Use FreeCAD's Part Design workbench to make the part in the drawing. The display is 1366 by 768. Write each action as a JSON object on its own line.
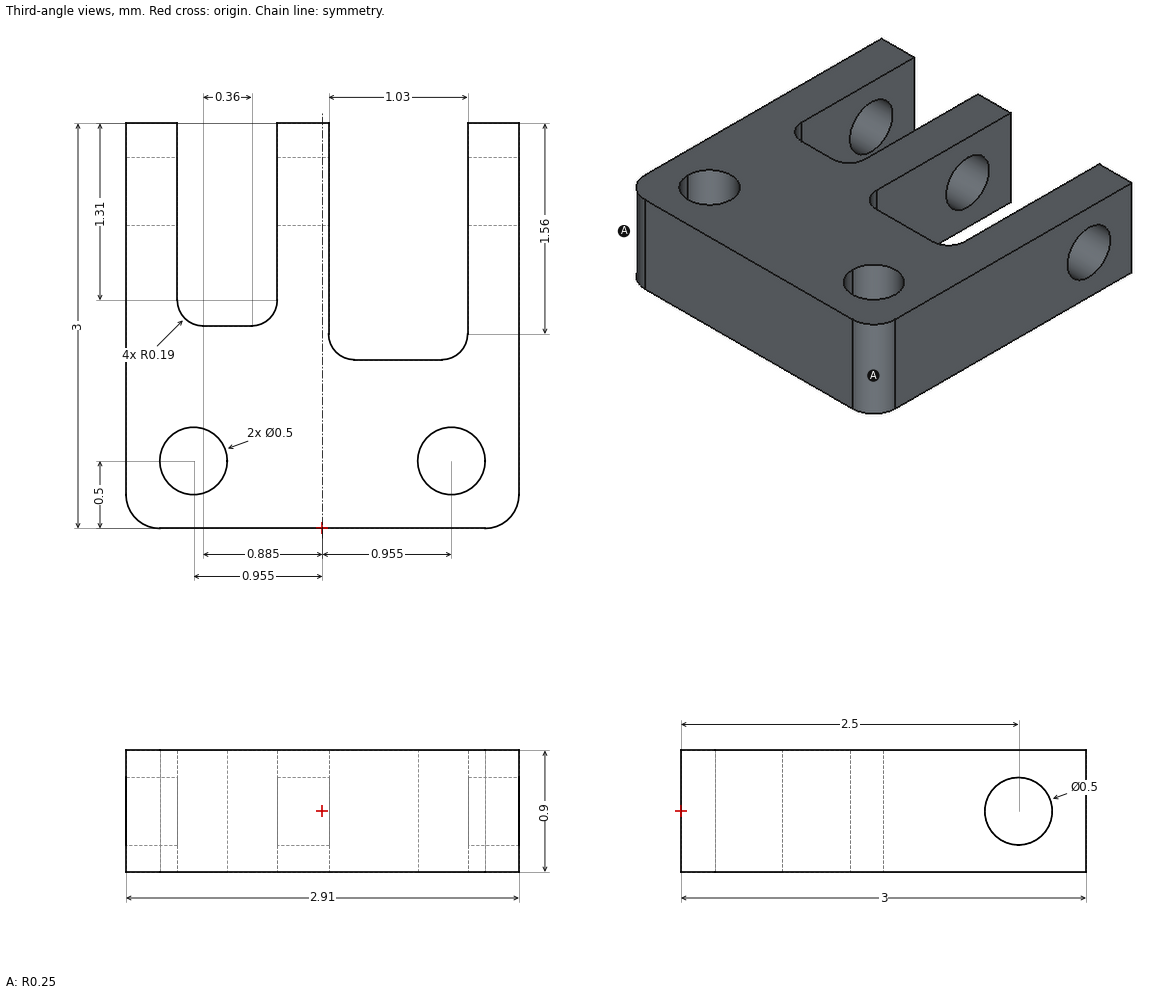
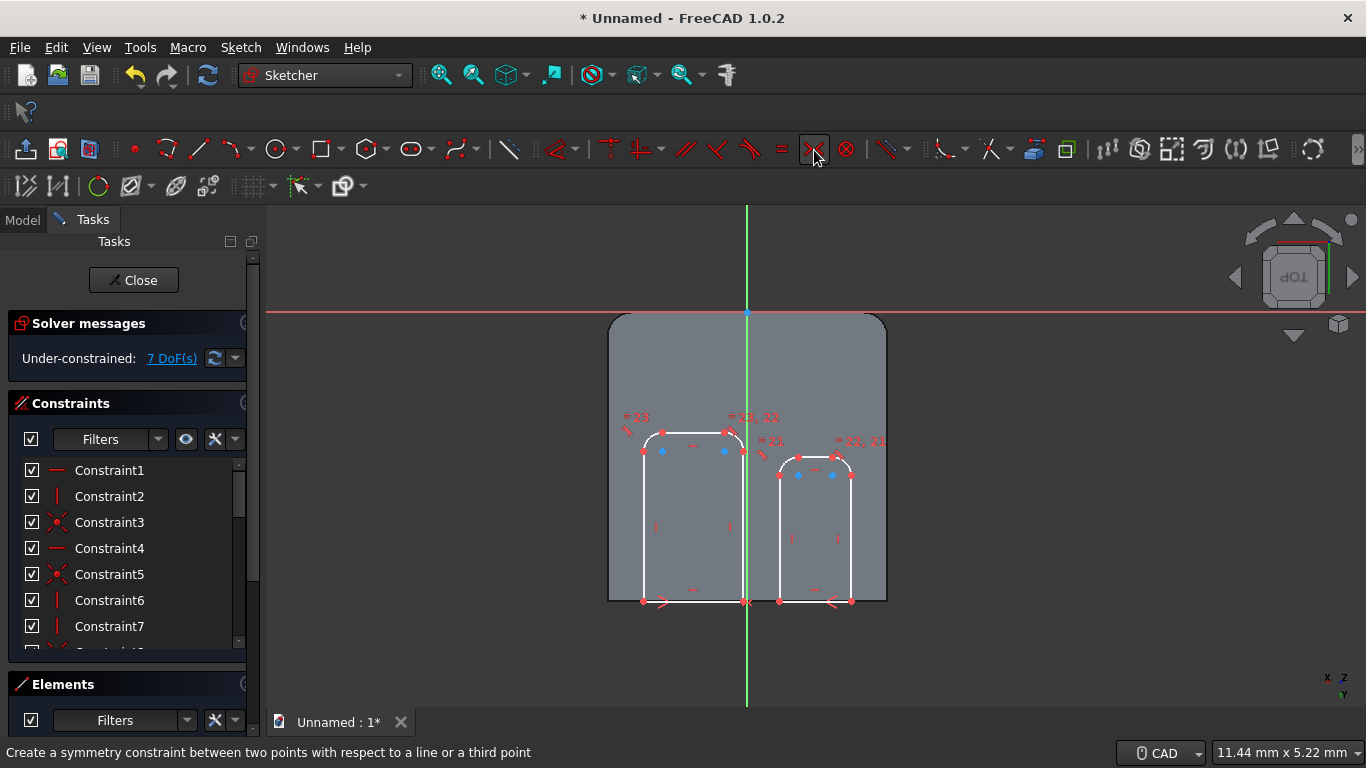
{"action": "scroll", "coordinate": [785, 463], "scroll_direction": "up", "scroll_amount": 4}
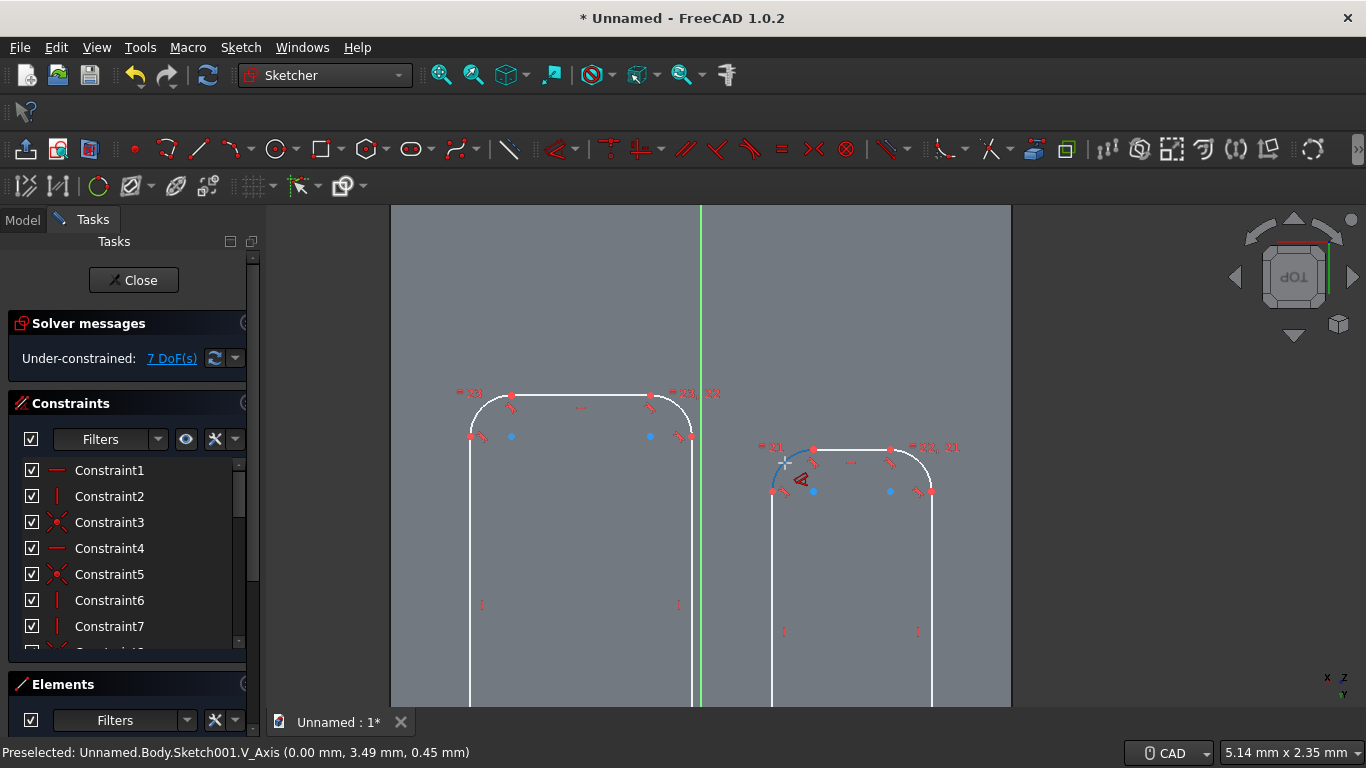
{"action": "left_click", "coordinate": [785, 462]}
{"action": "left_click", "coordinate": [763, 439]}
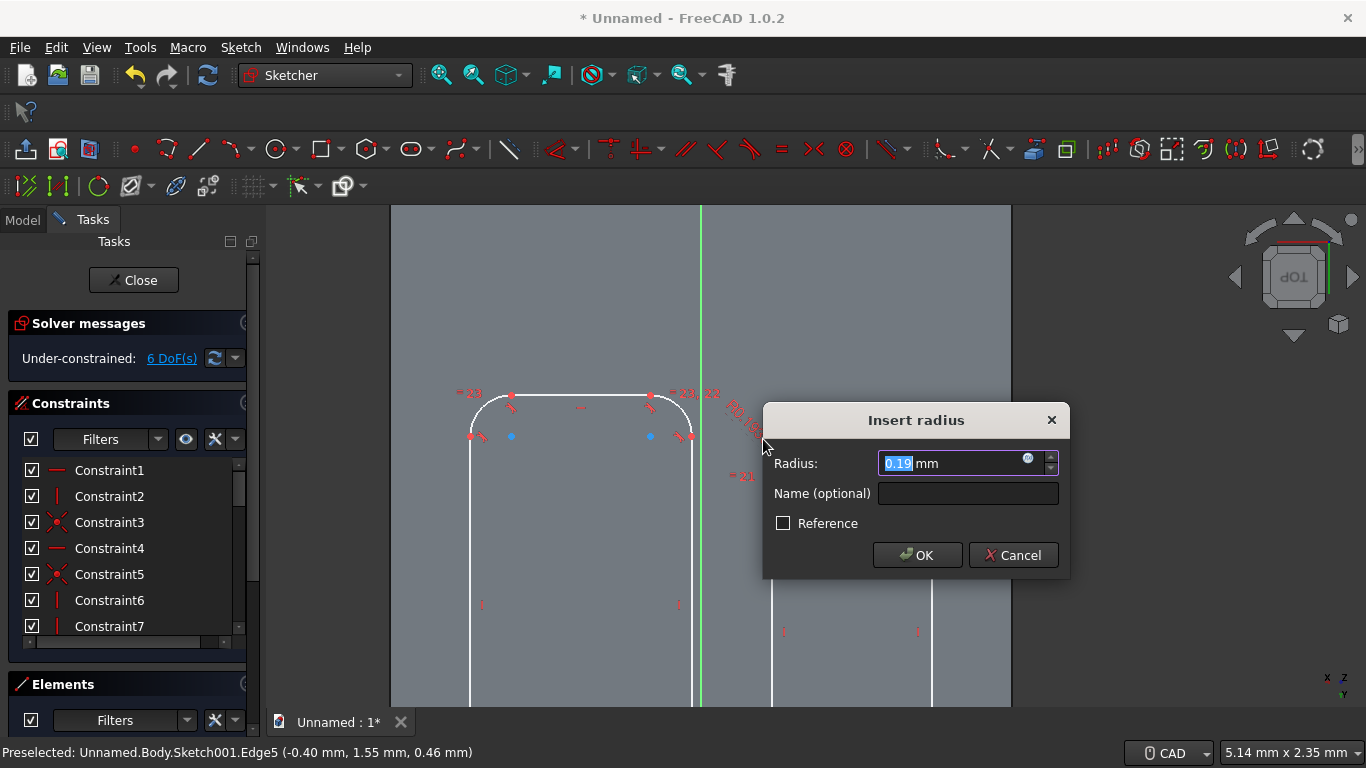
{"action": "type", "text": "0.19"}
{"action": "key", "text": "Return"}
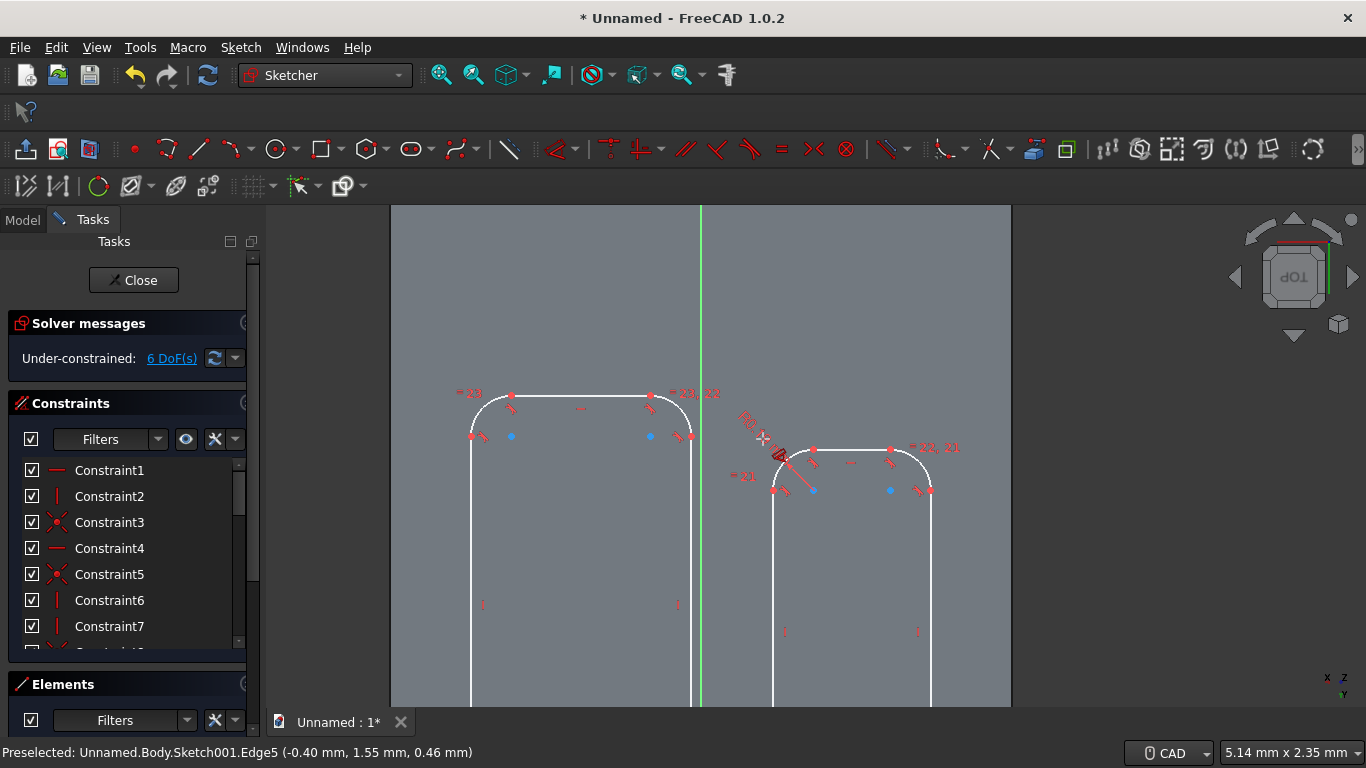
{"action": "scroll", "coordinate": [785, 462], "scroll_direction": "down", "scroll_amount": 4}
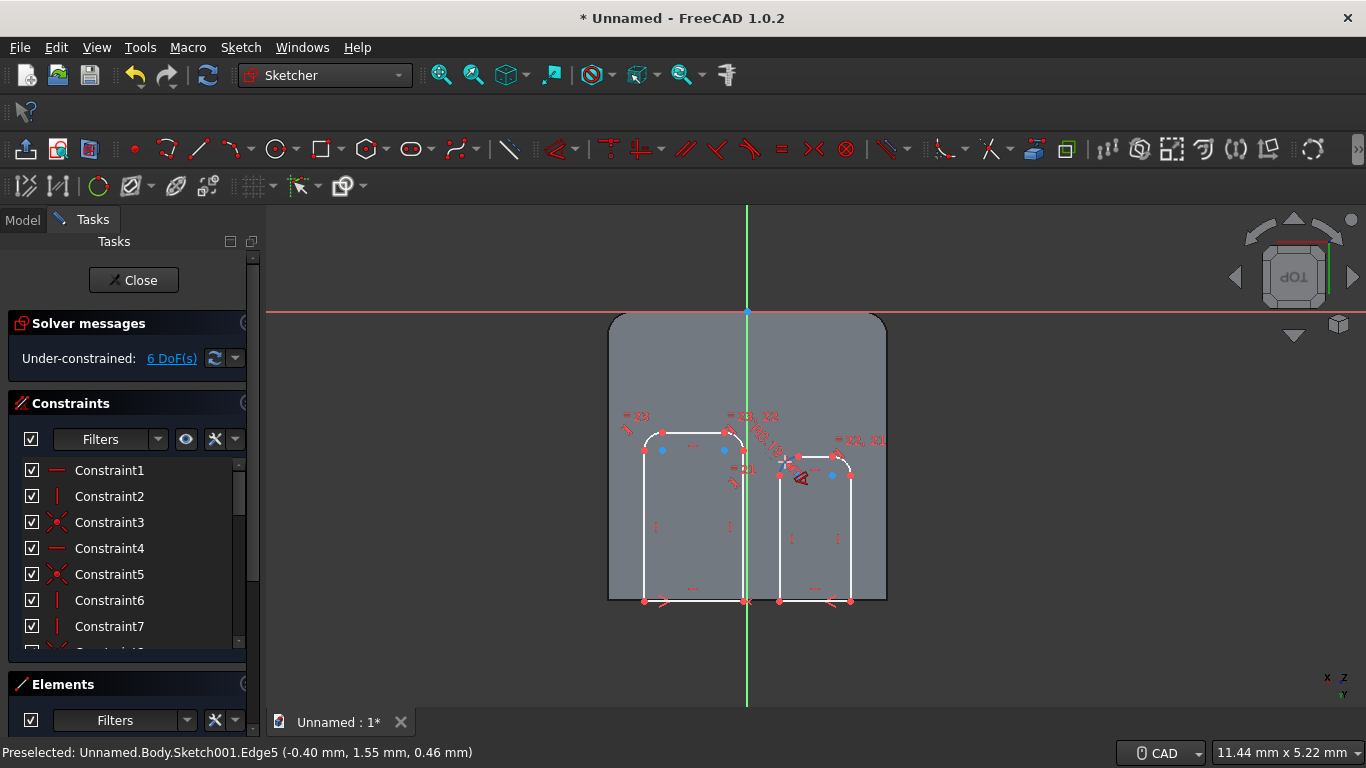
{"action": "left_click", "coordinate": [780, 601]}
{"action": "left_click", "coordinate": [814, 390]}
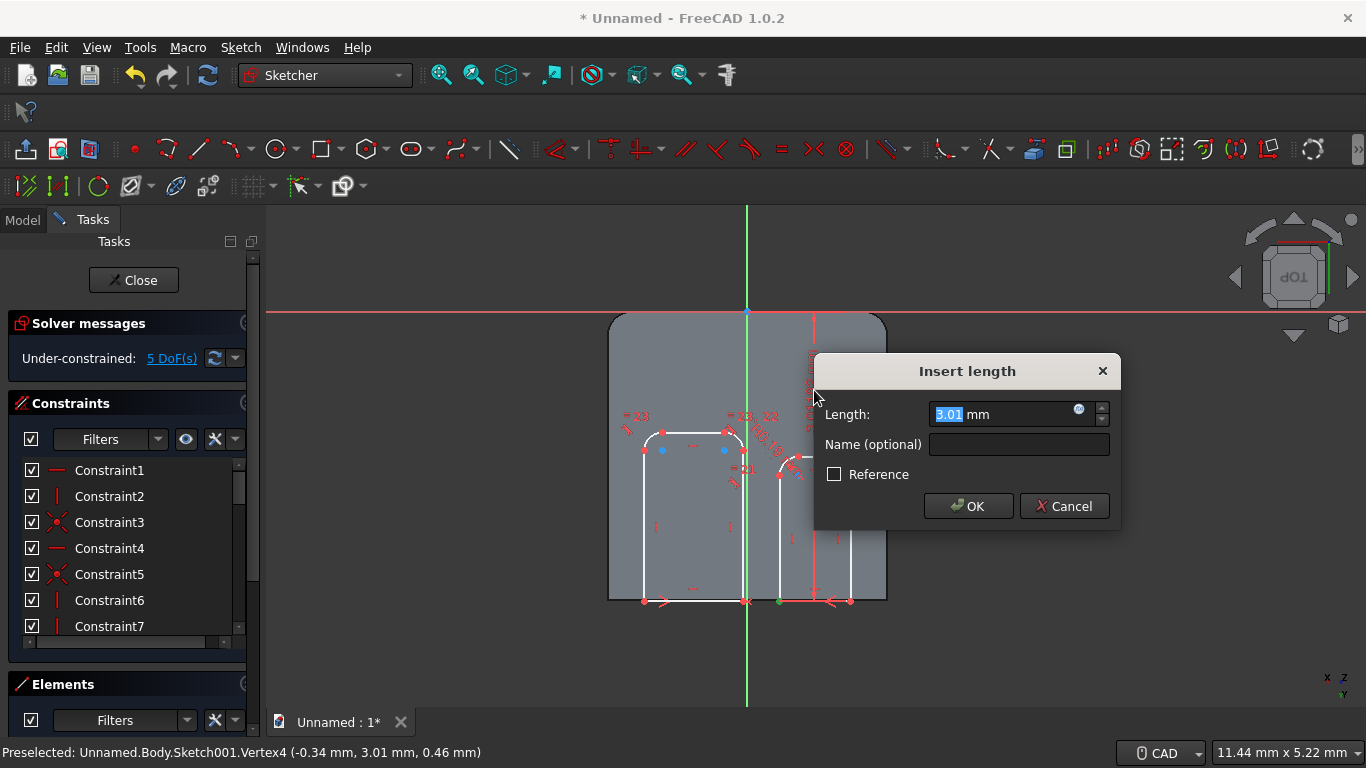
{"action": "type", "text": "3"}
{"action": "key", "text": "Return"}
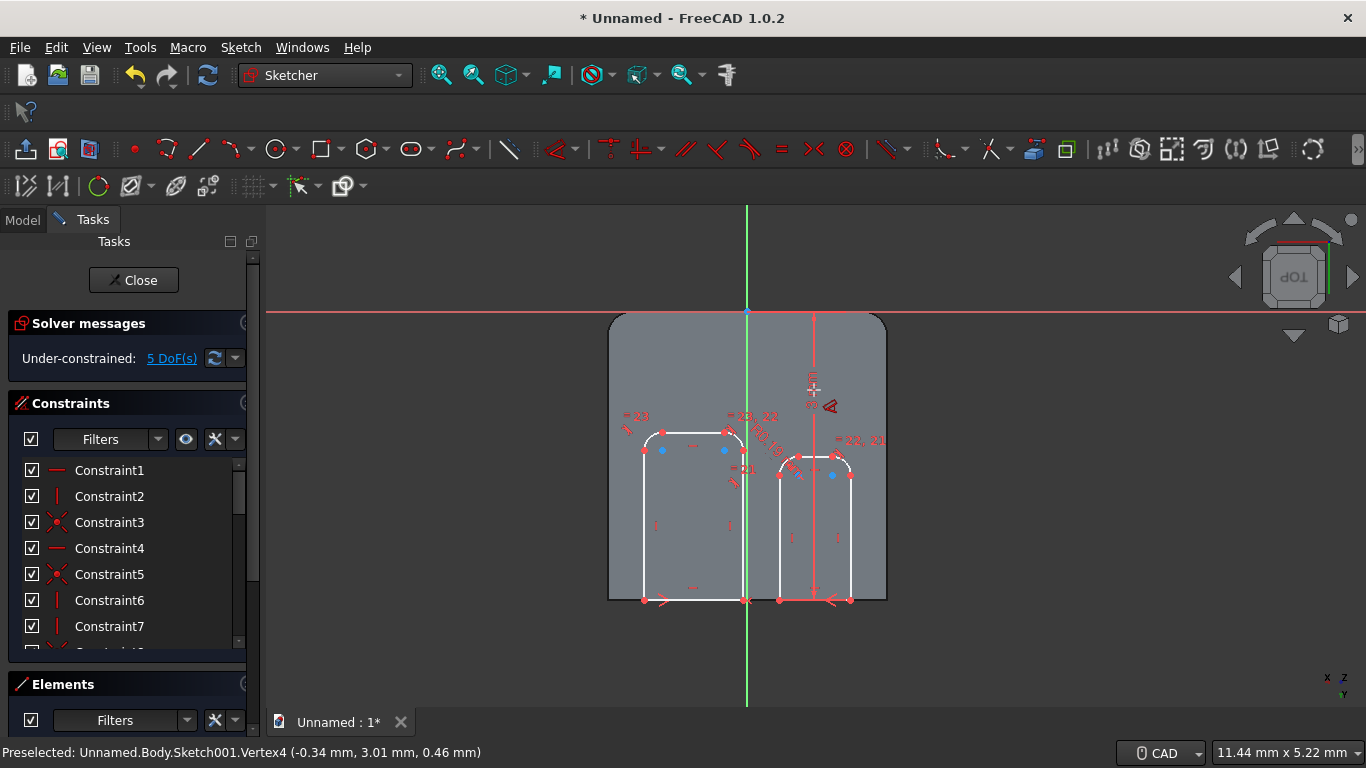
{"action": "scroll", "coordinate": [822, 457], "scroll_direction": "up", "scroll_amount": 2}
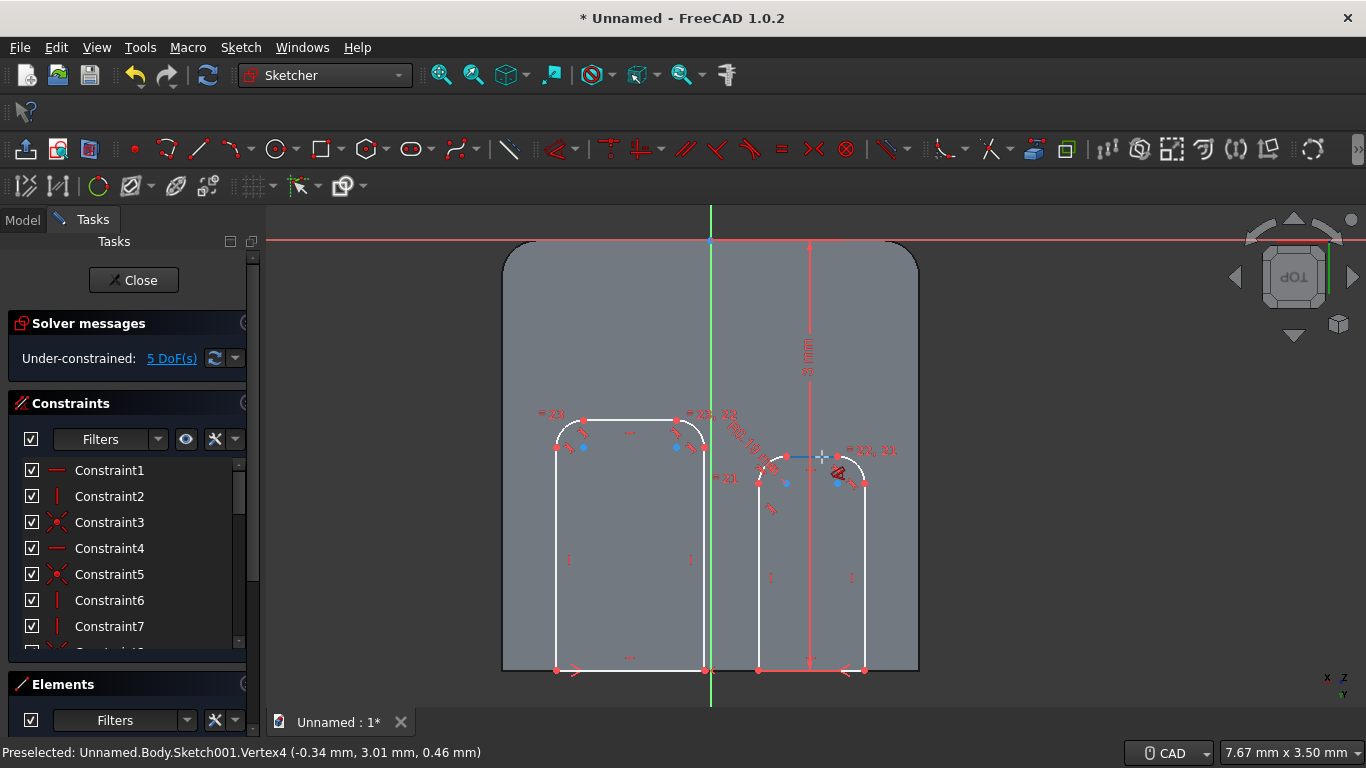
{"action": "left_click", "coordinate": [822, 457]}
{"action": "left_click", "coordinate": [812, 491]}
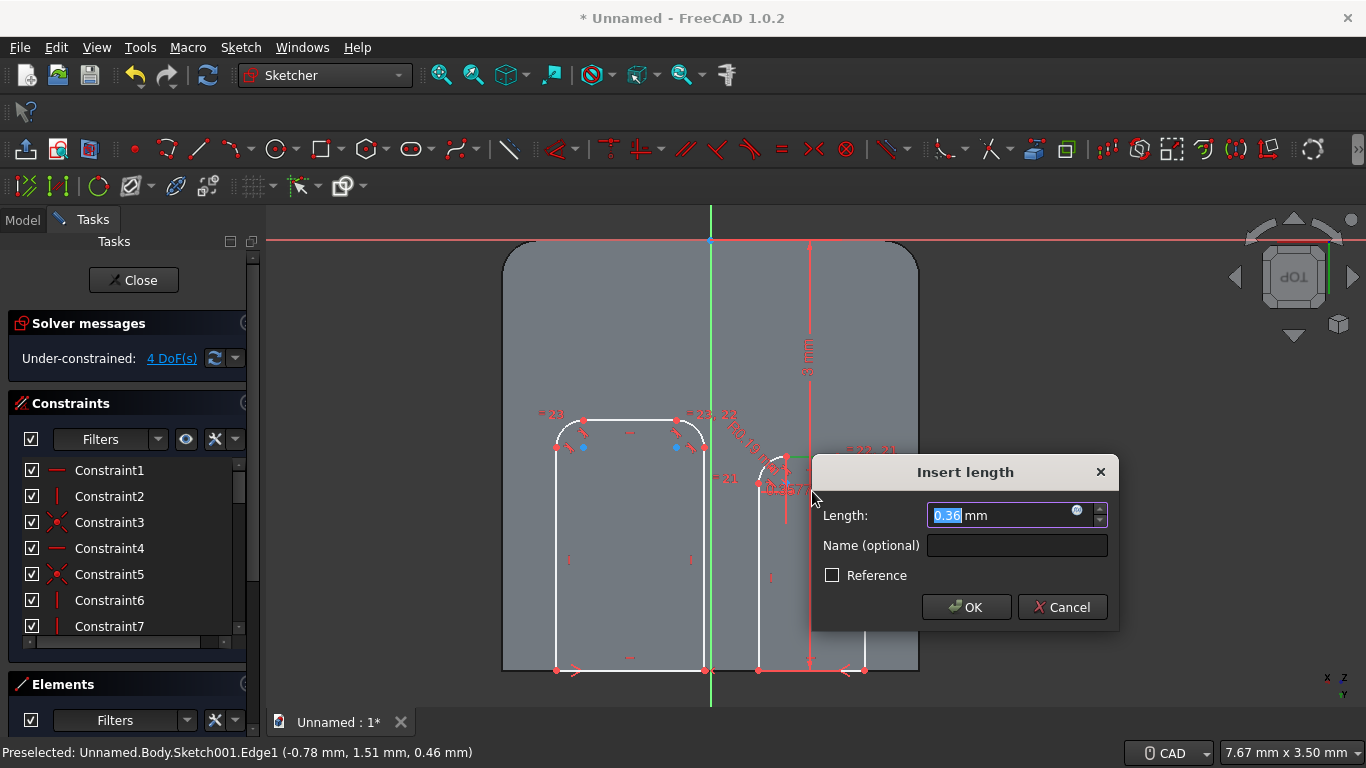
{"action": "type", "text": "0.36"}
{"action": "key", "text": "Return"}